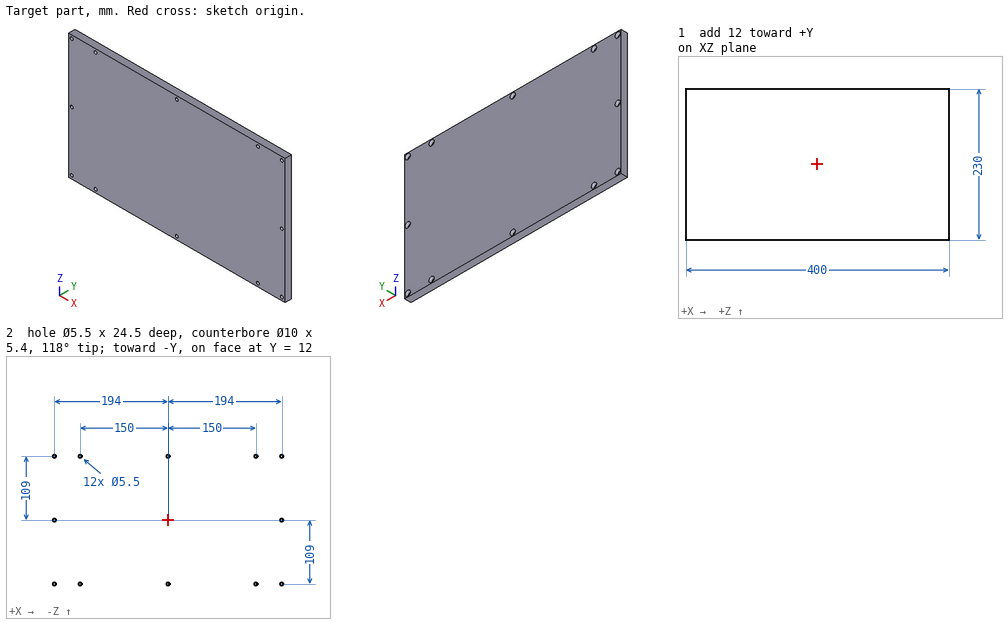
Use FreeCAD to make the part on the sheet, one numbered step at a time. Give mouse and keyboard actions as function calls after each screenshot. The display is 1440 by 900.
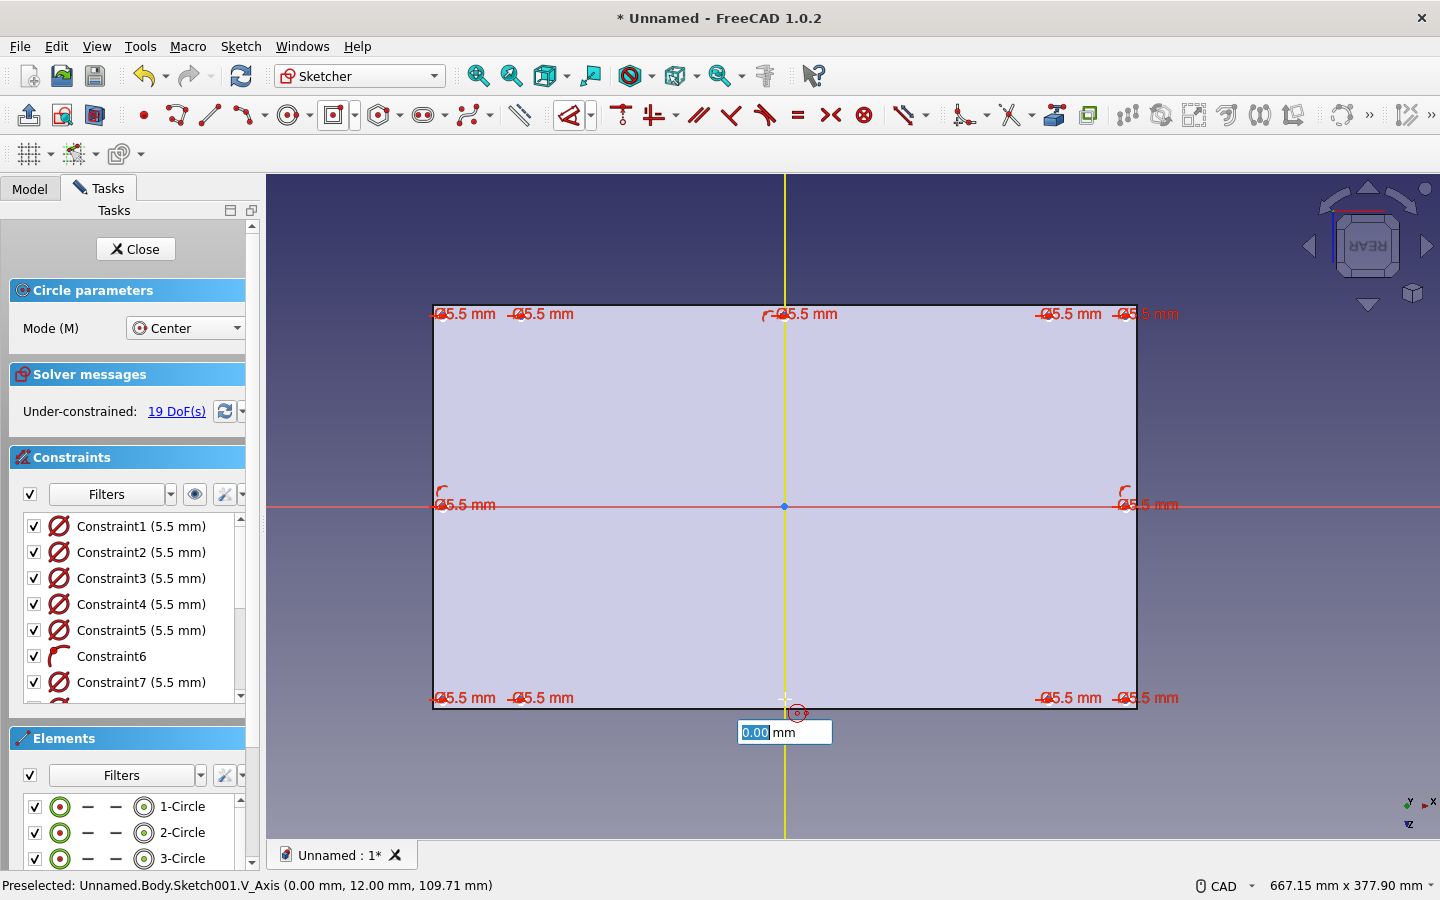
scroll(789, 697, up, 7)
move(789, 695)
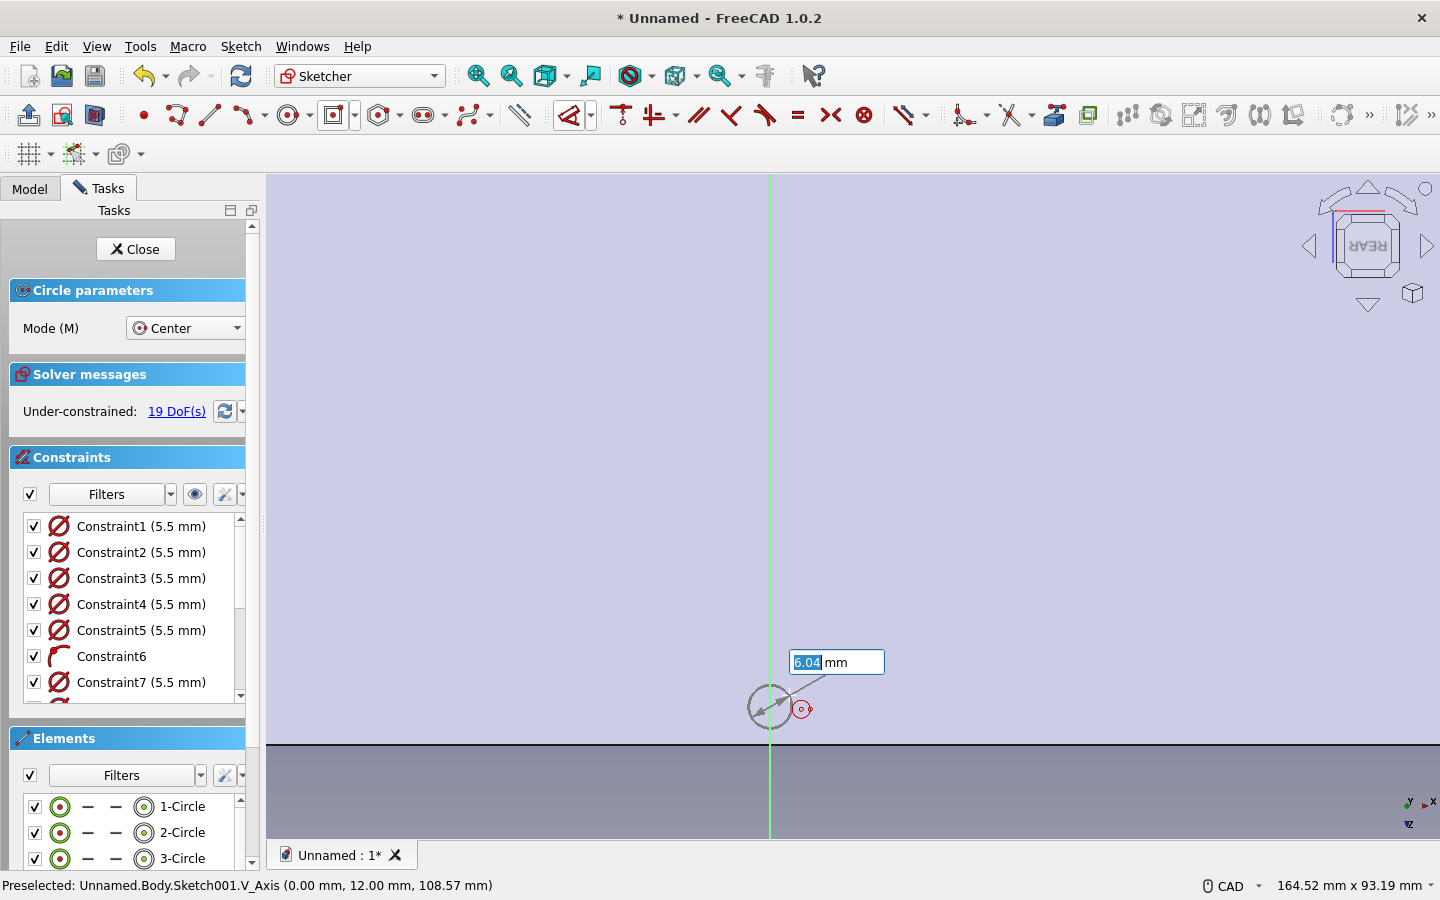
text(5.5)
key(Return)
key(Escape)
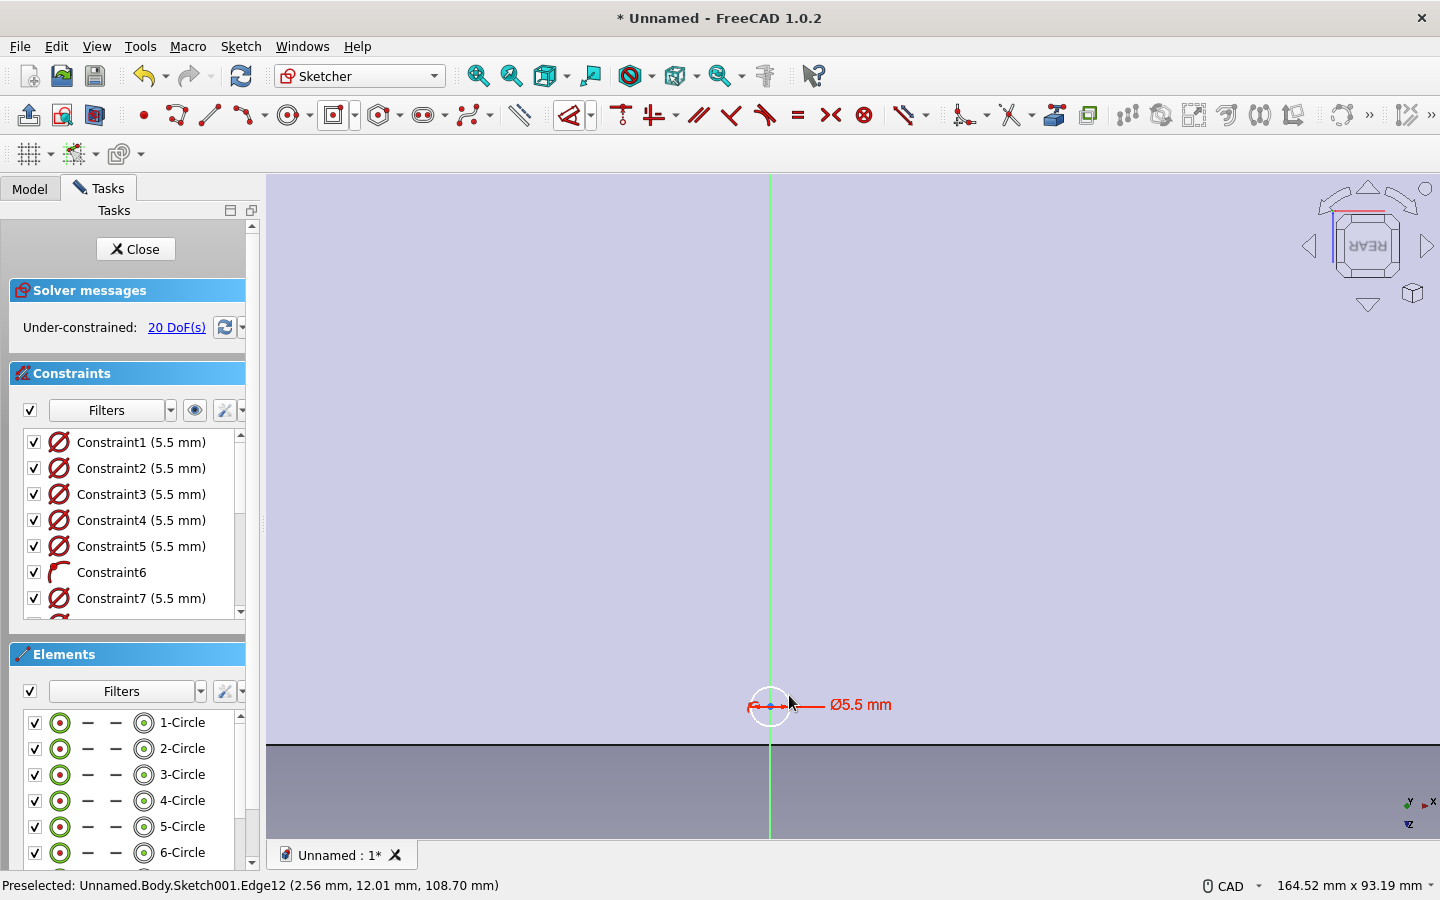
scroll(789, 697, down, 7)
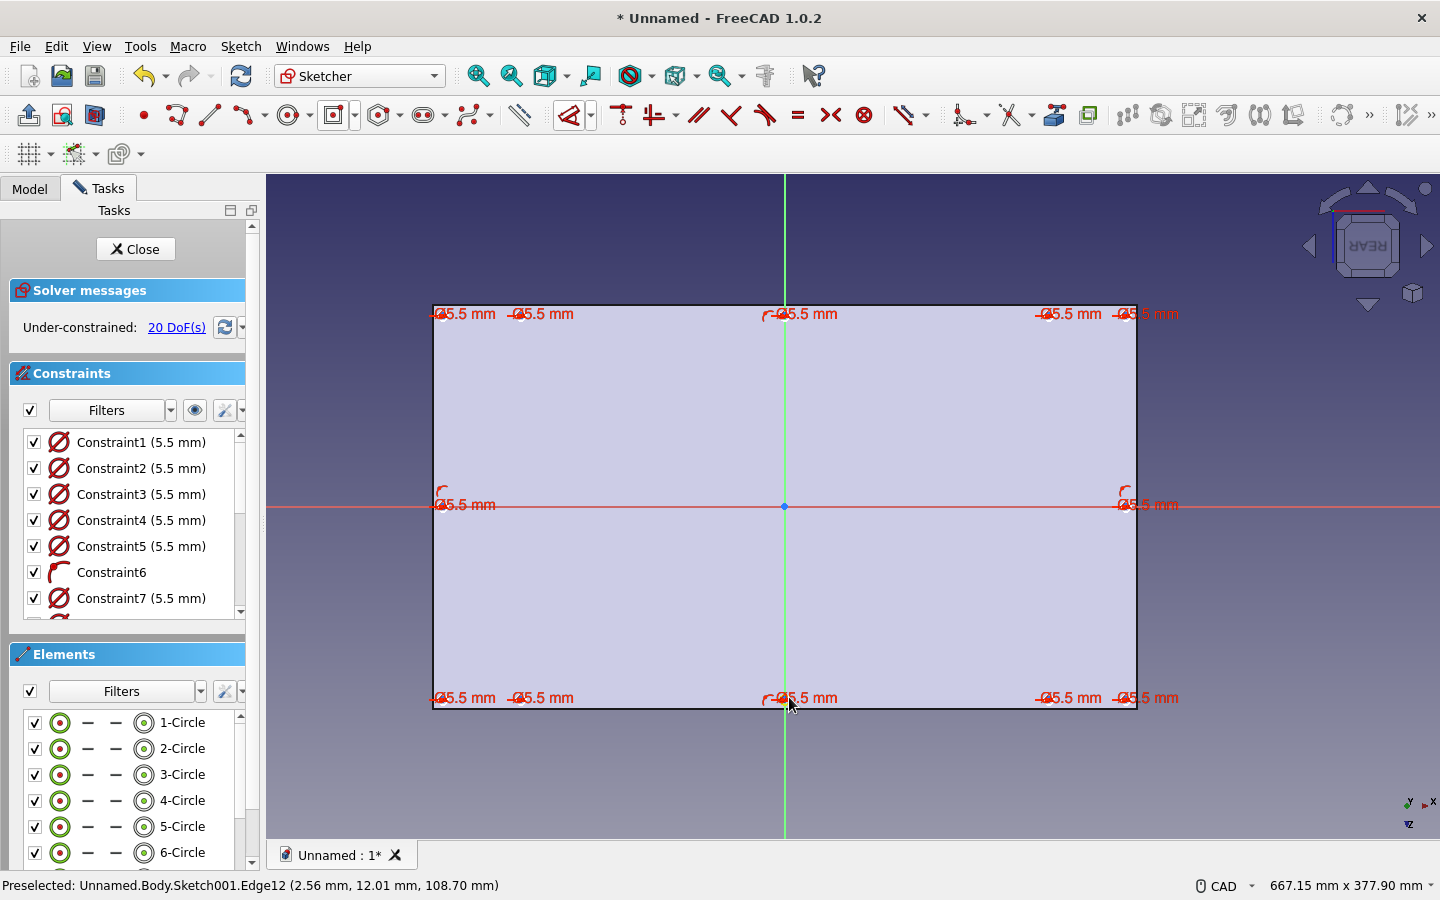
click(443, 316)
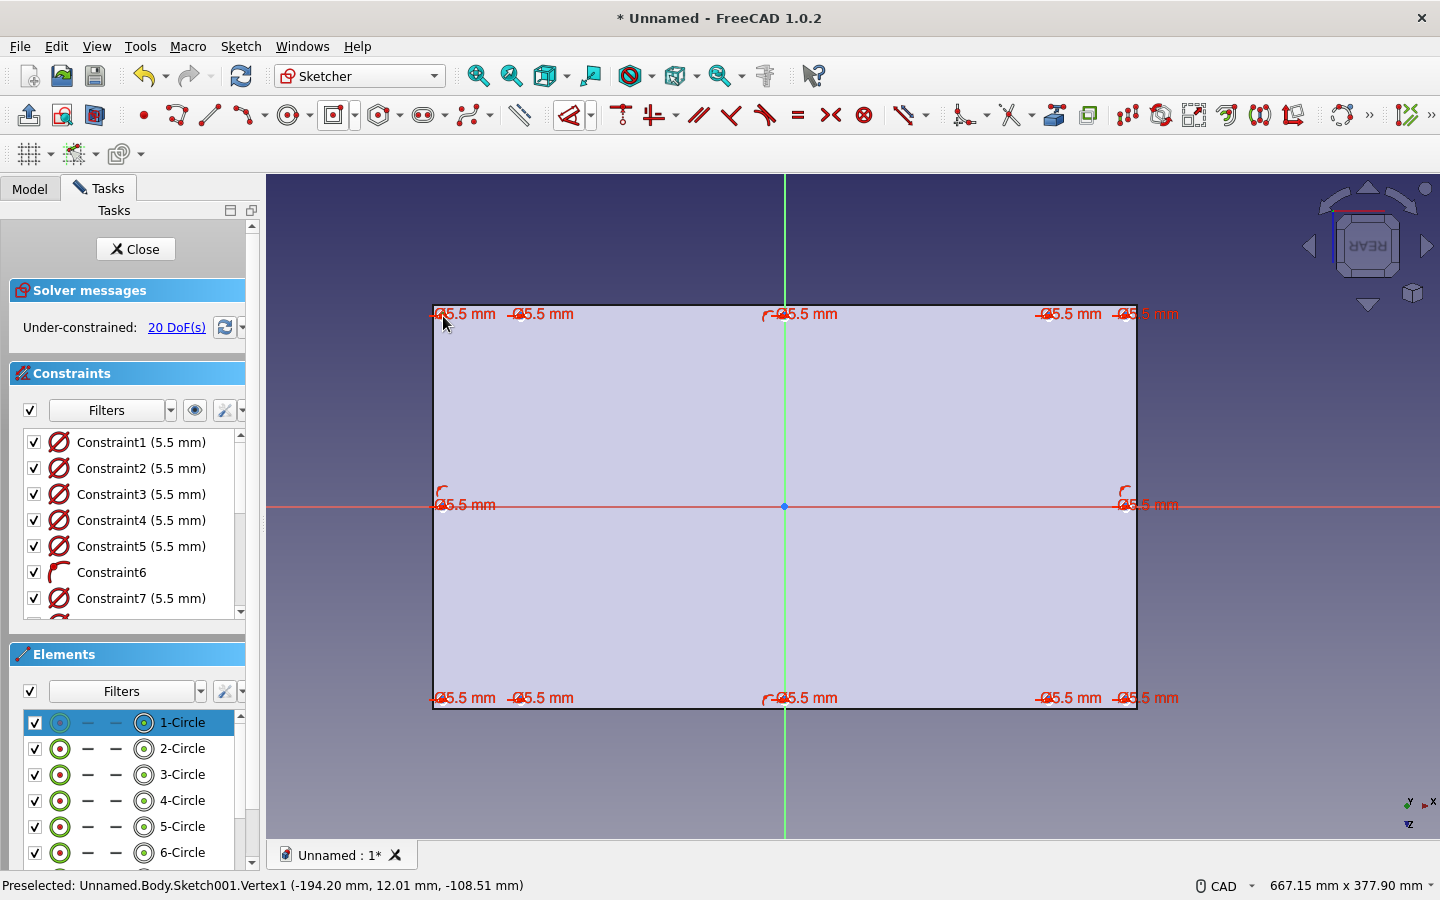
click(521, 316)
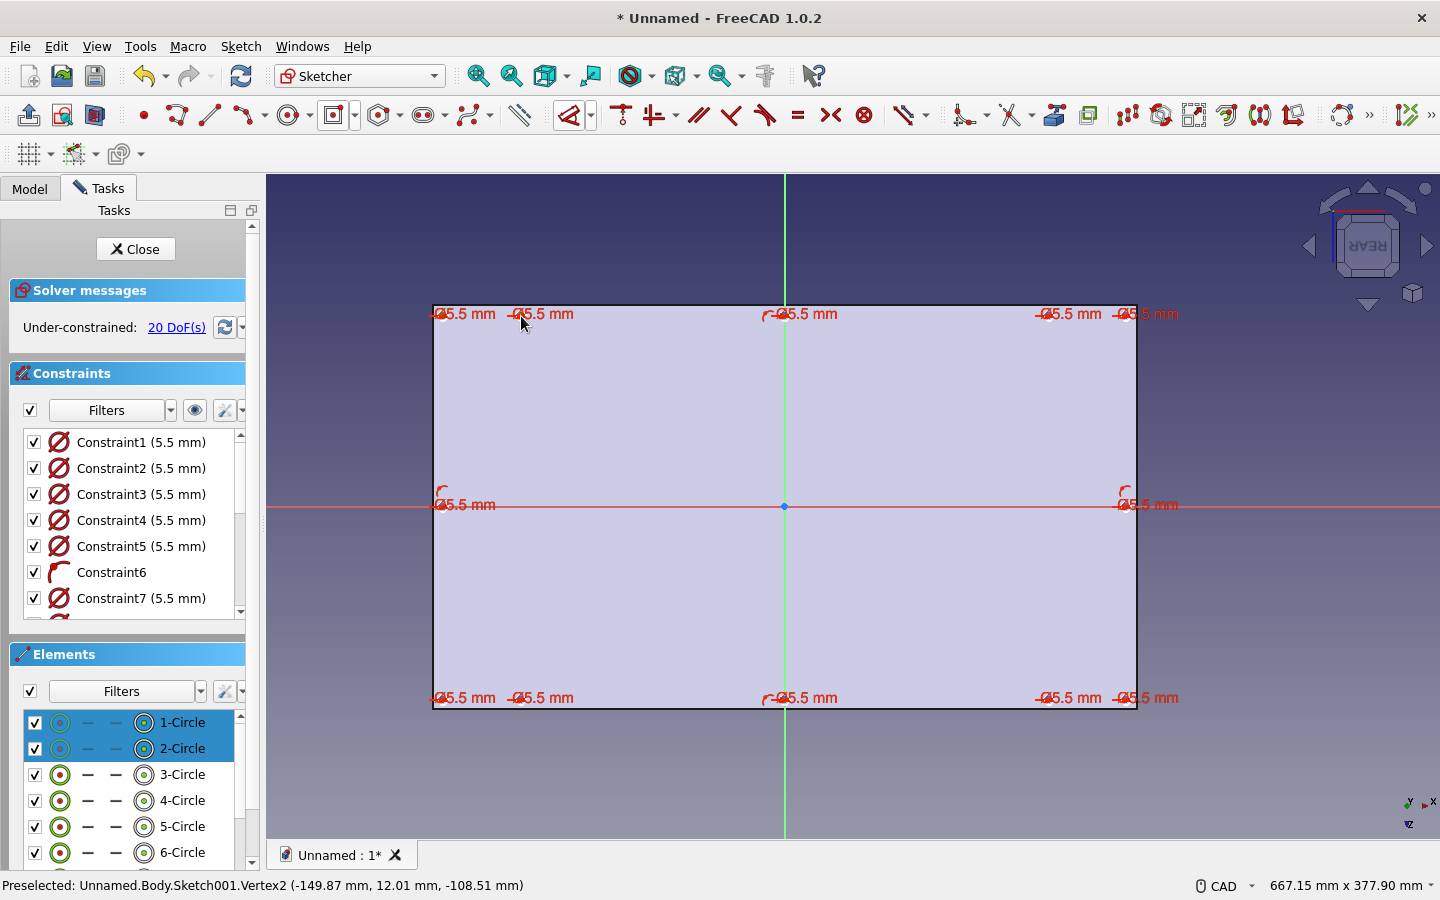
click(676, 116)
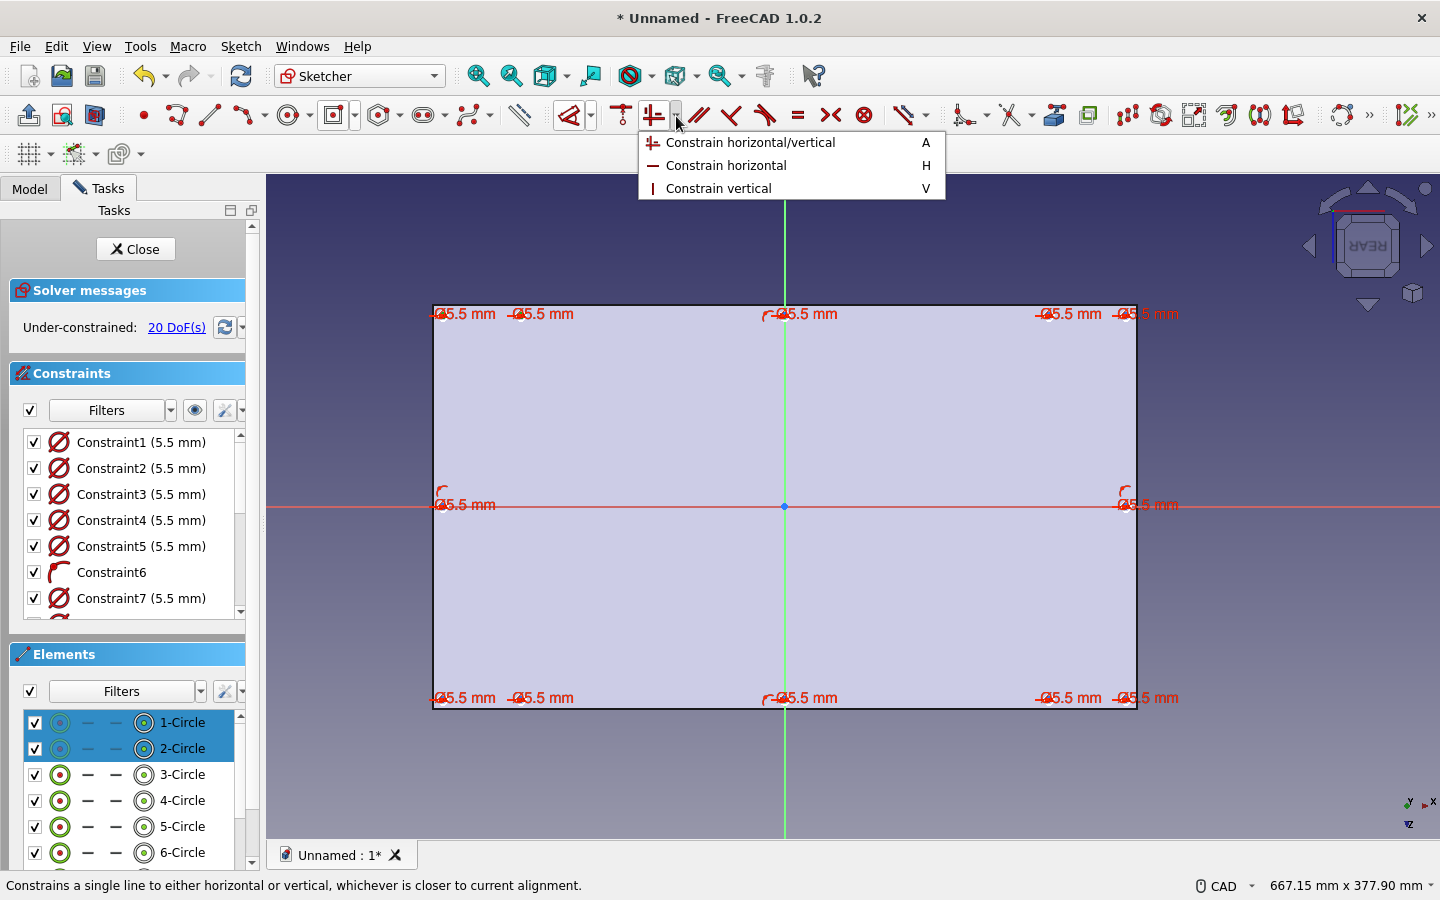
click(792, 166)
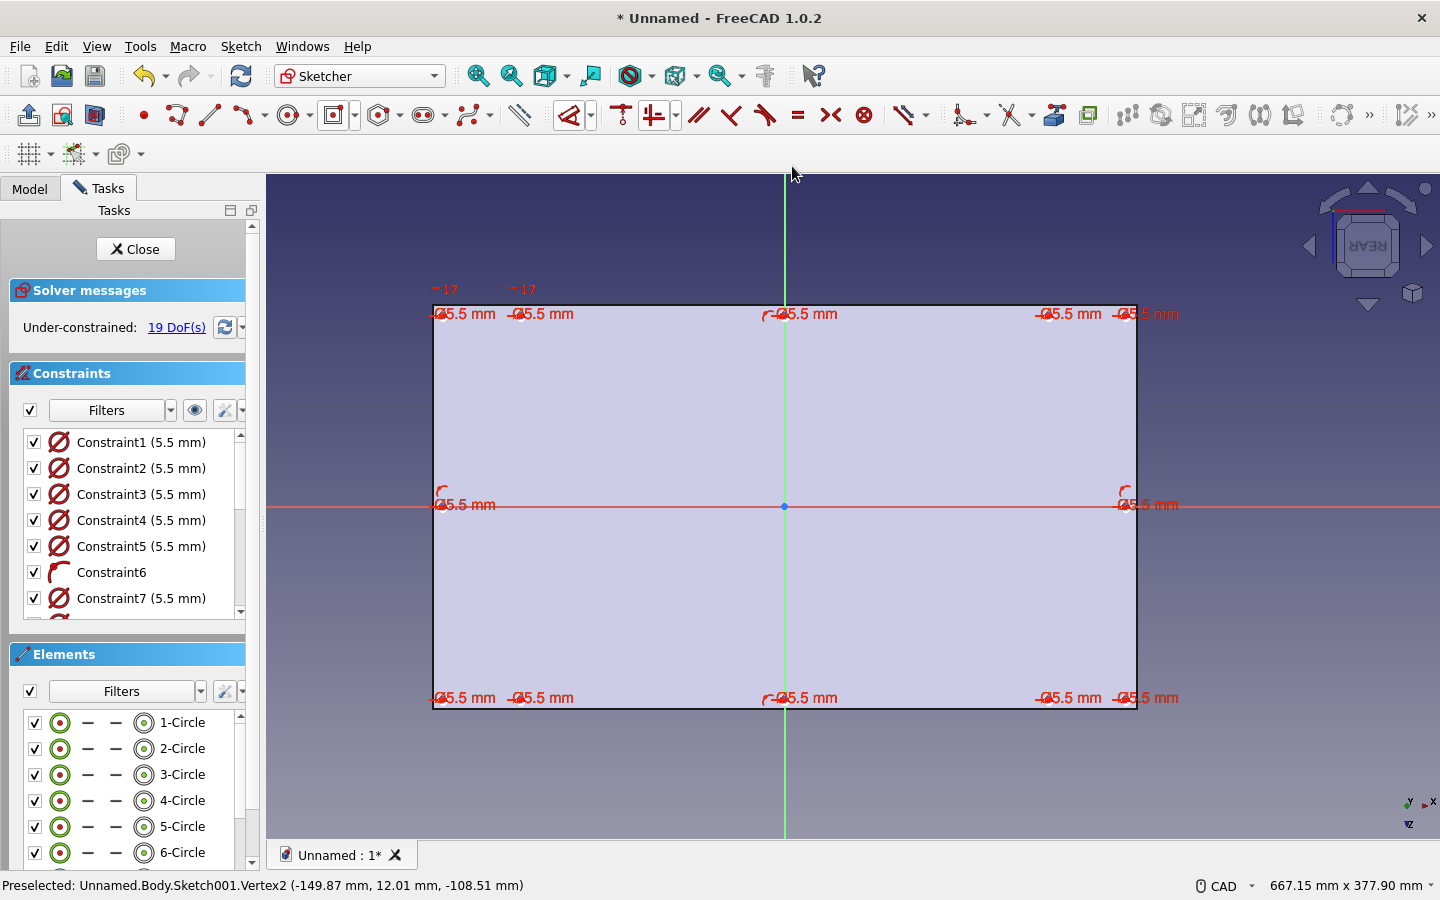
click(521, 316)